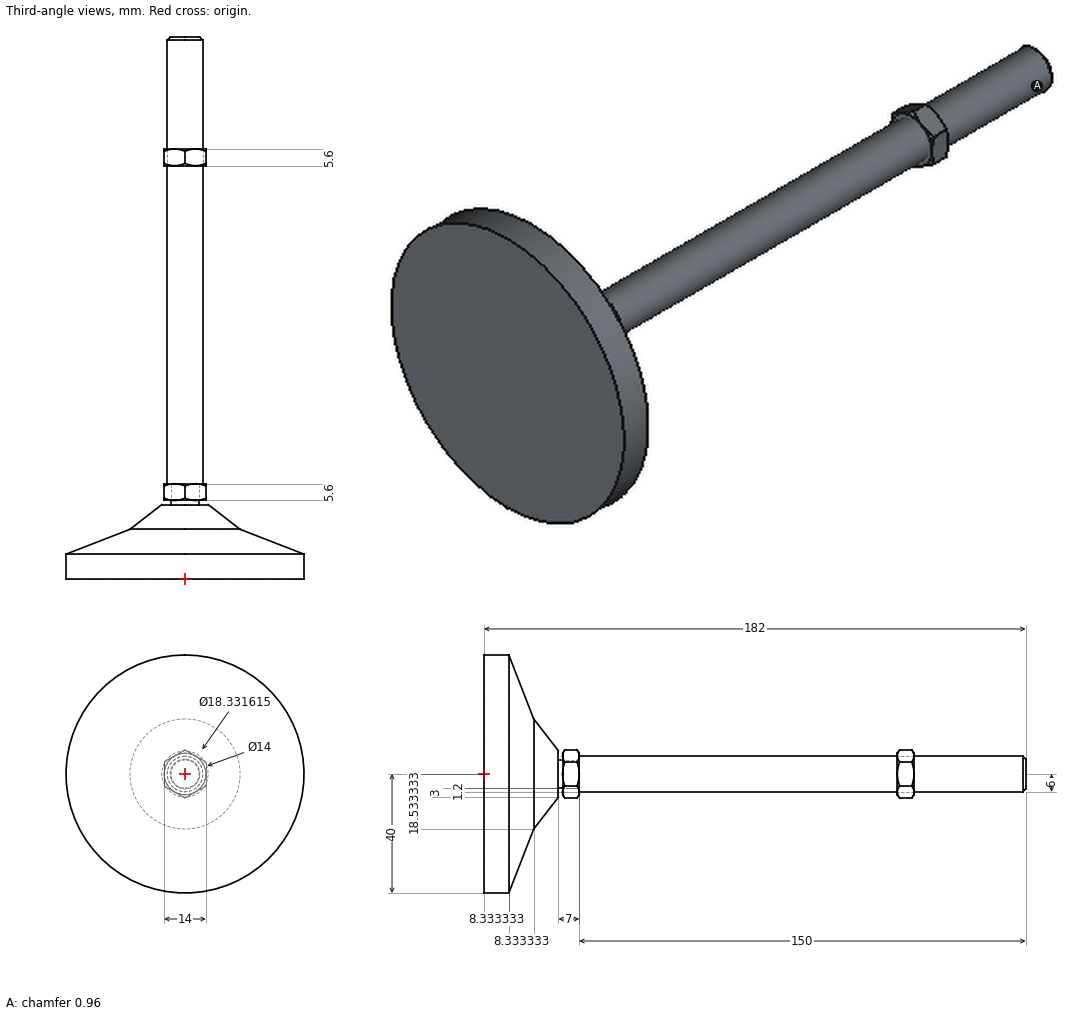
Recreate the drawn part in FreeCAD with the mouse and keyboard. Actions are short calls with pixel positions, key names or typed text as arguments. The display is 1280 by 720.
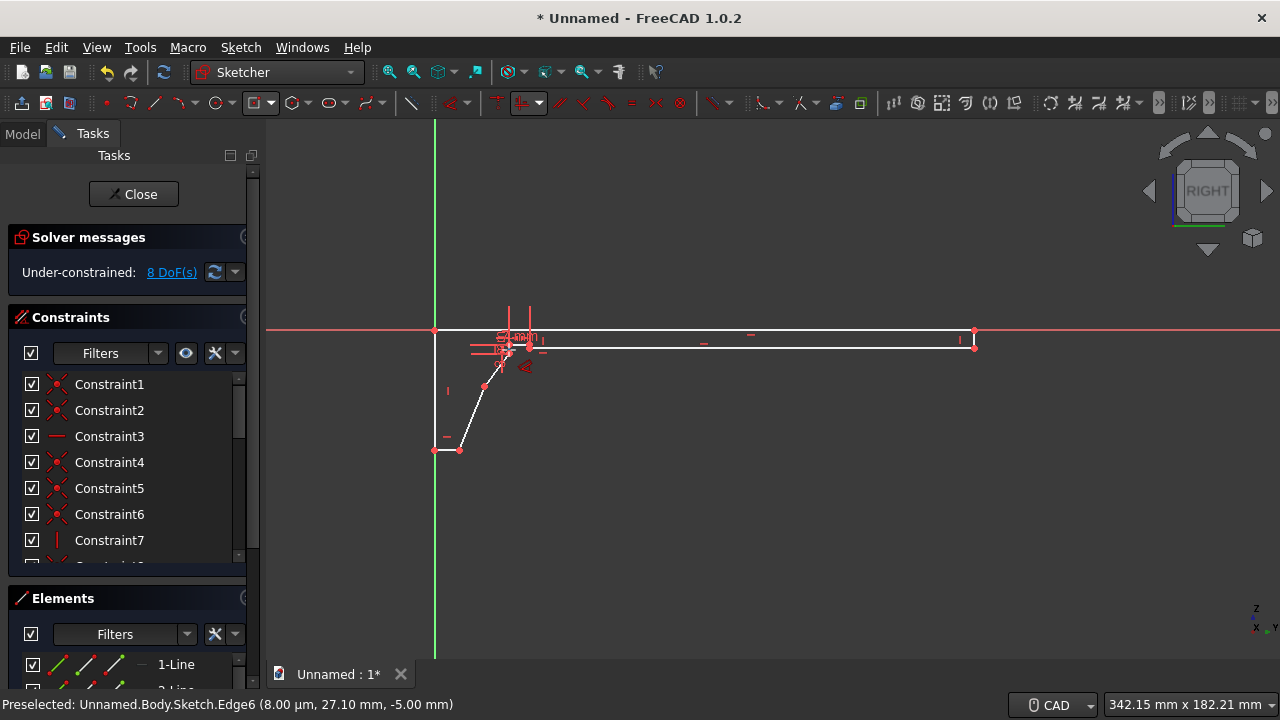
scroll(974, 343, up, 5)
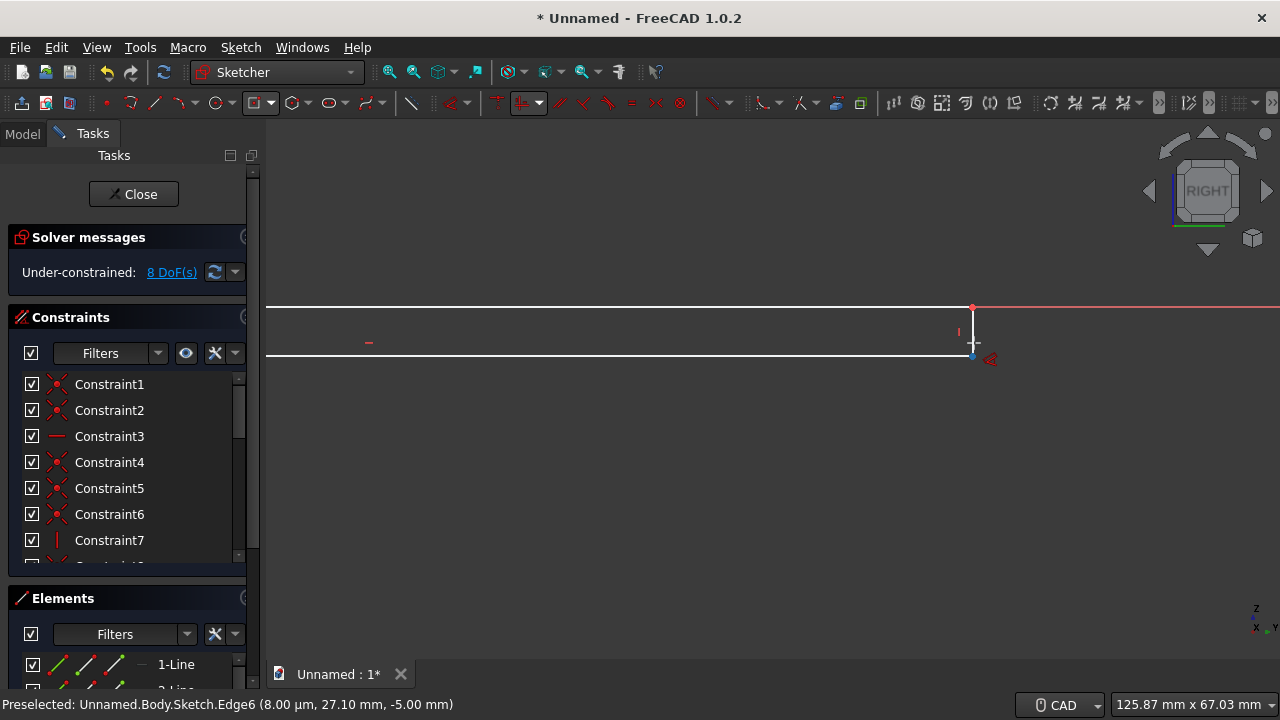
click(973, 342)
click(1007, 332)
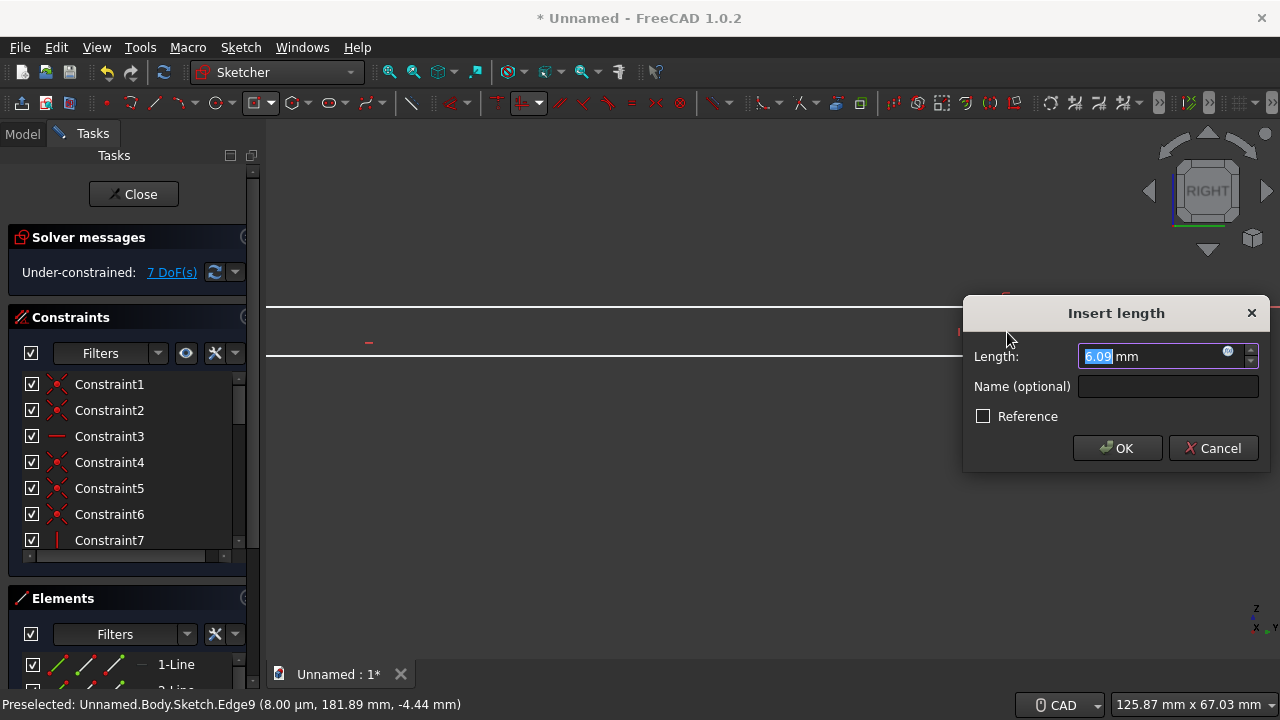
text(6)
key(Return)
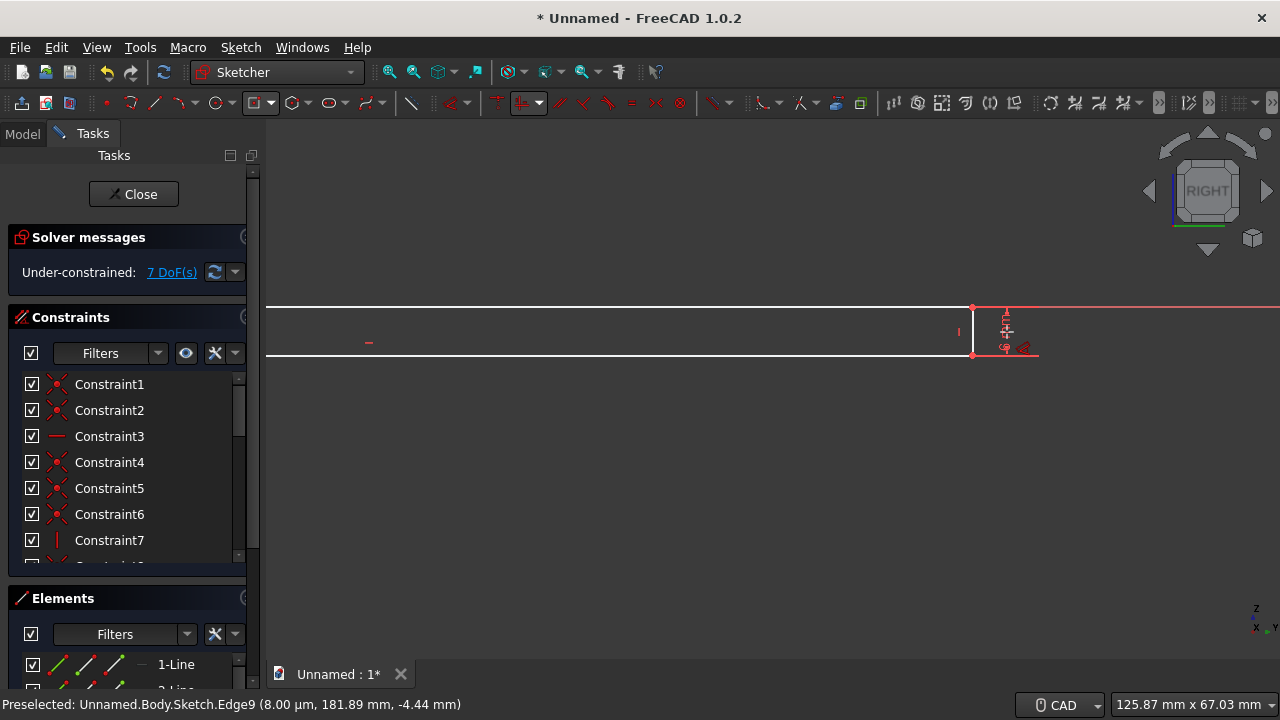
scroll(974, 343, down, 5)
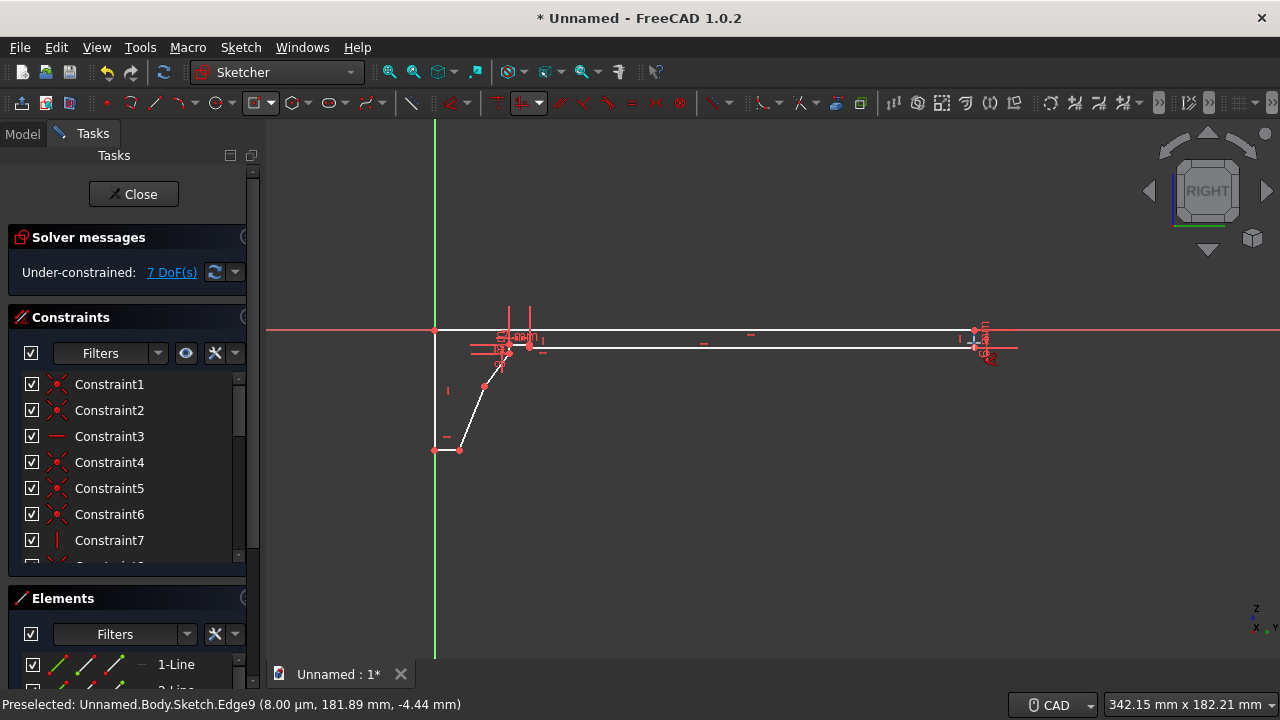
click(435, 366)
click(401, 390)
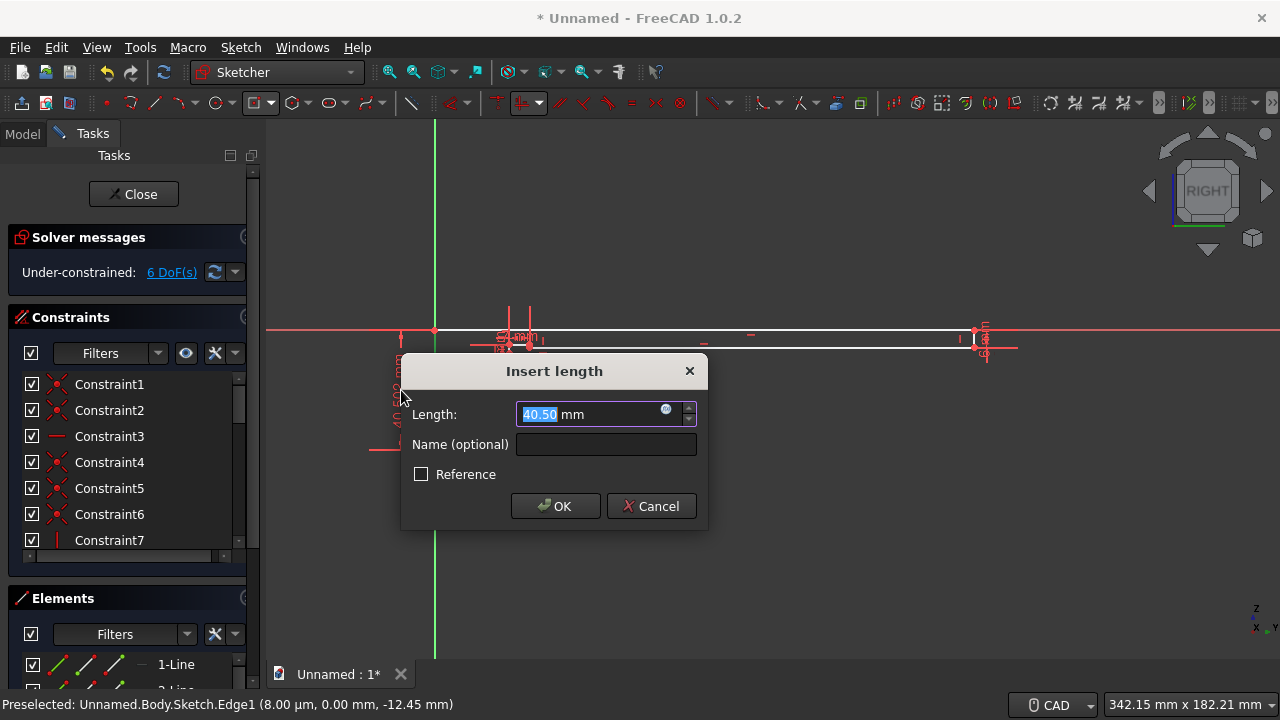
text(40)
key(Return)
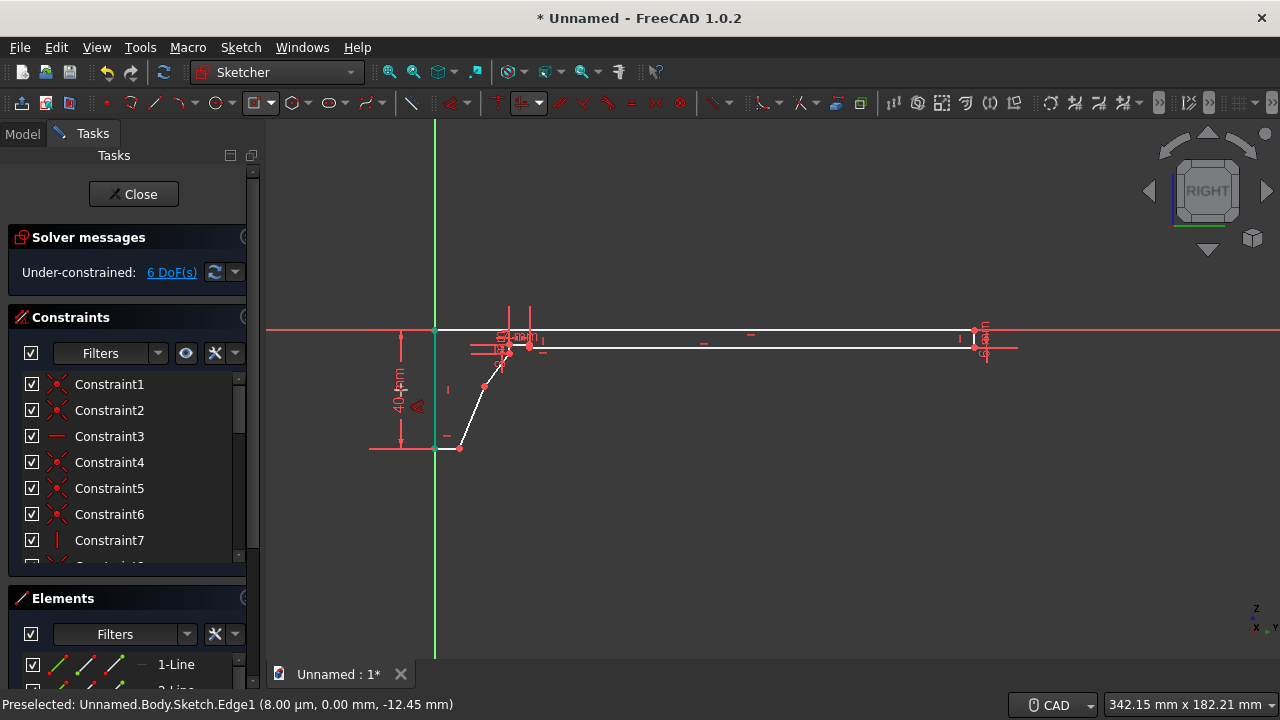
scroll(530, 346, up, 13)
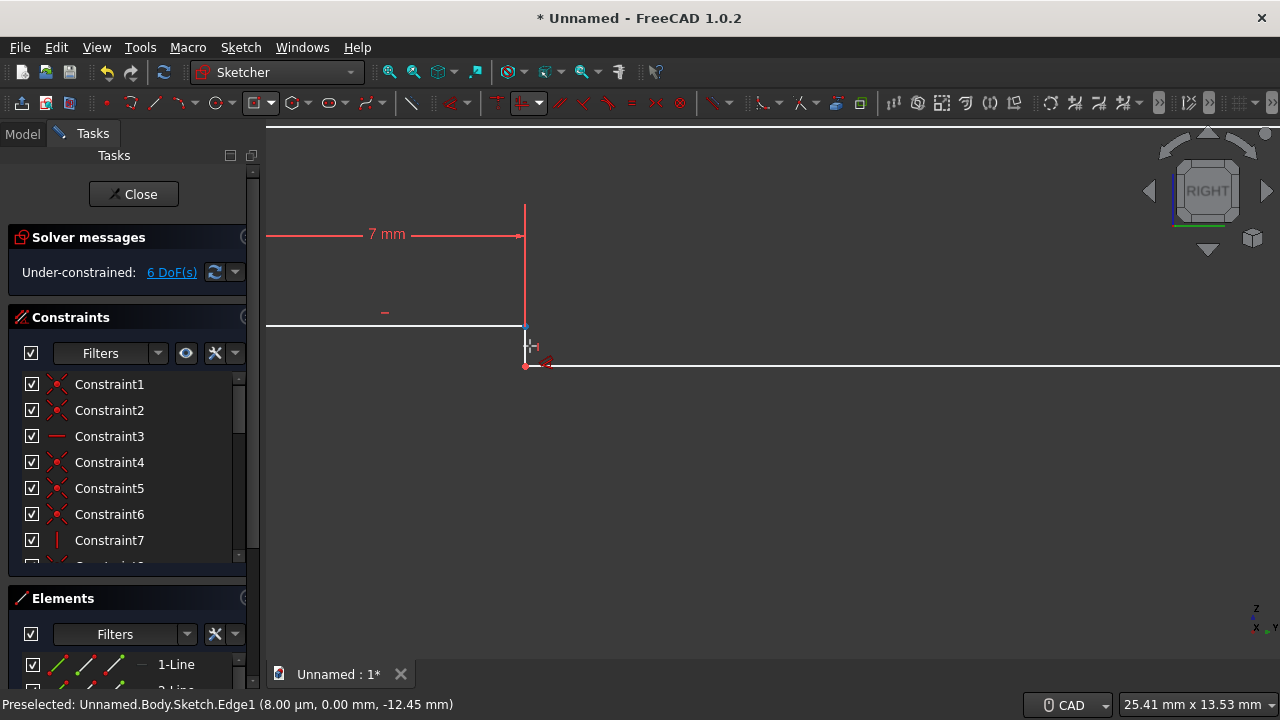
click(525, 346)
click(491, 346)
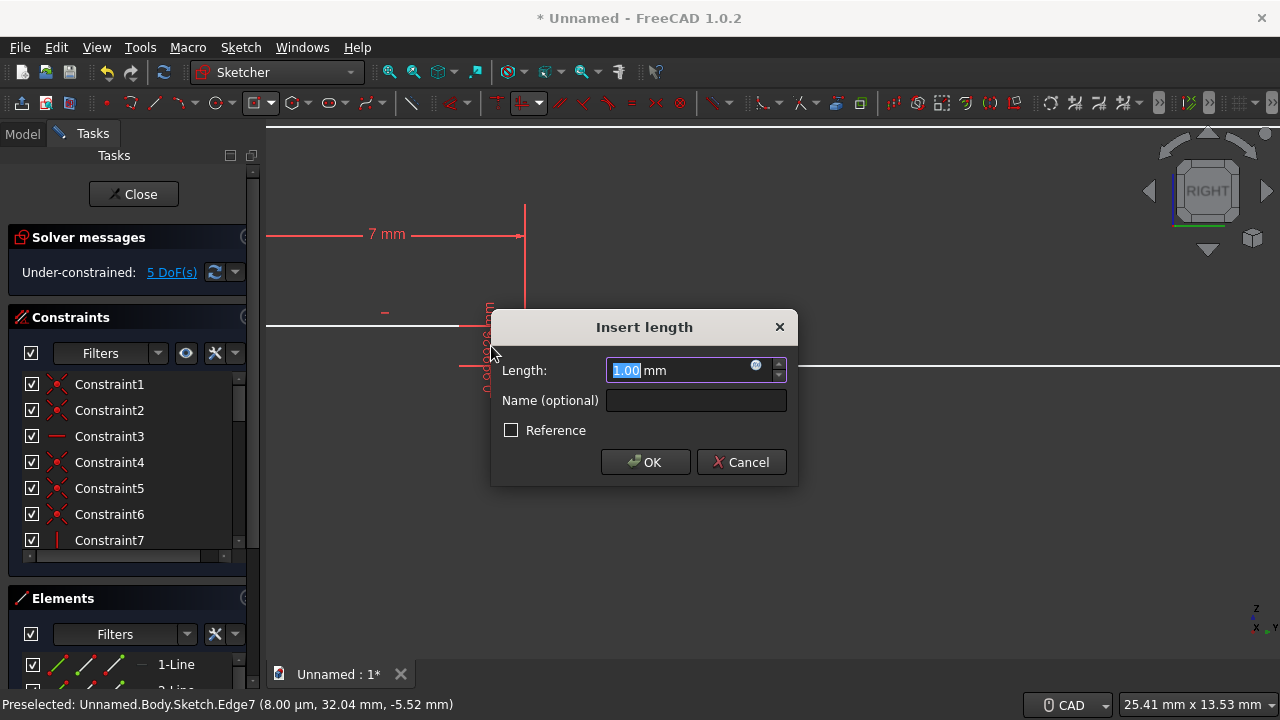
text(1.2)
key(Return)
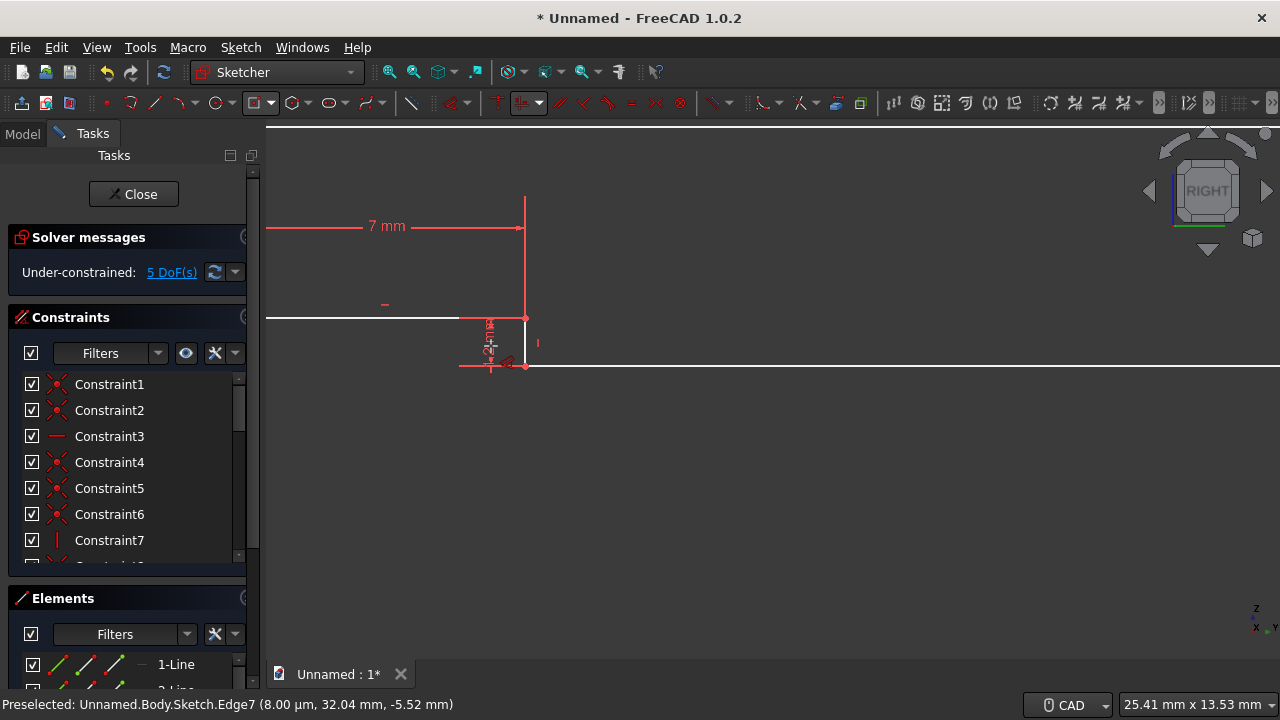
scroll(530, 346, down, 13)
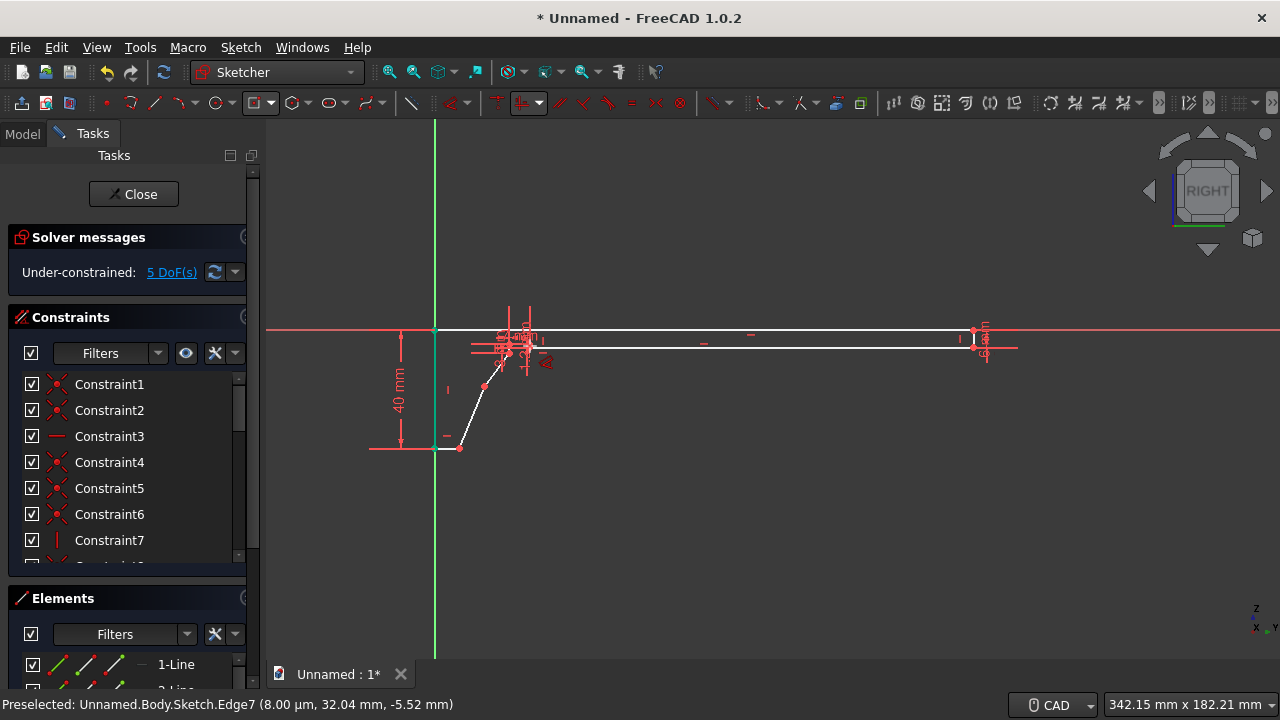
click(663, 348)
click(752, 314)